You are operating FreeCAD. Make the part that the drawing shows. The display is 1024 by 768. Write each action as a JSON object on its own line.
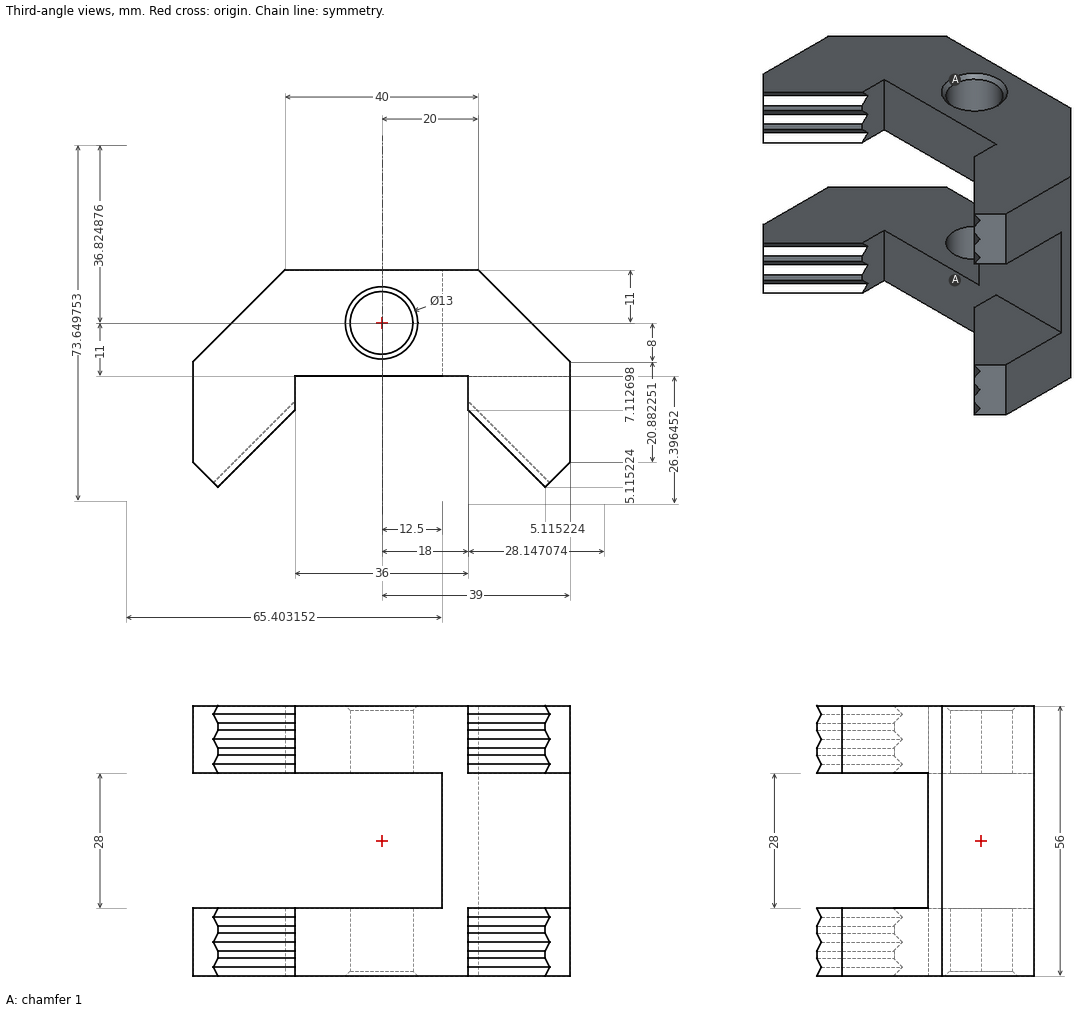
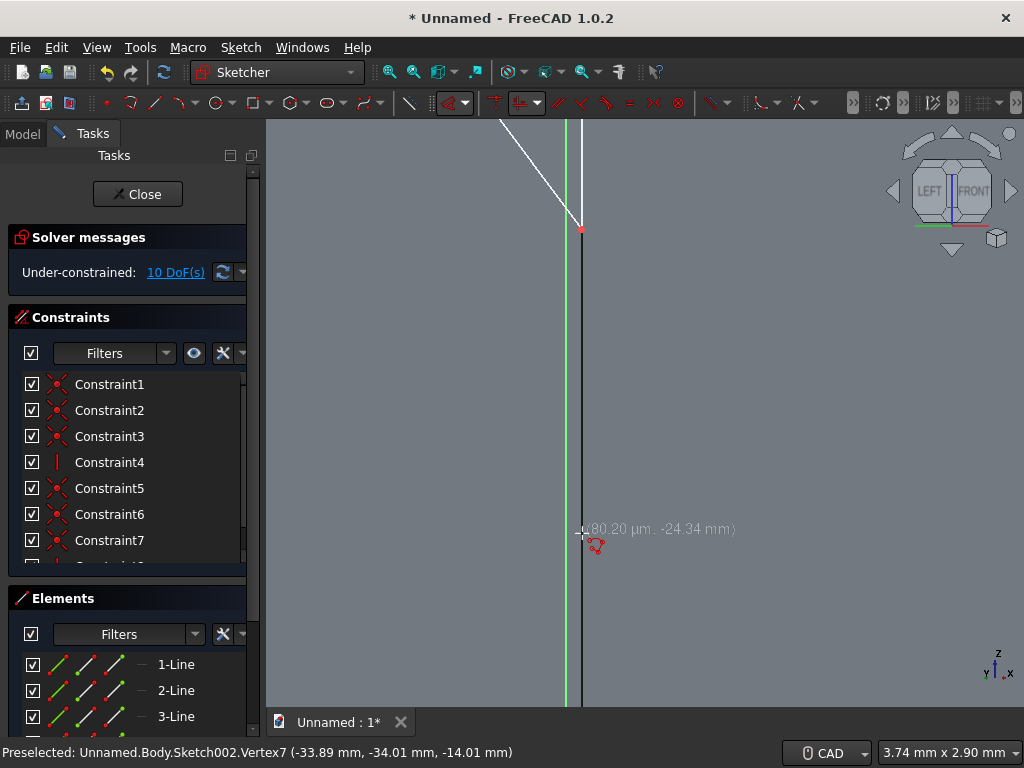
{"action": "scroll", "coordinate": [585, 541], "scroll_direction": "down", "scroll_amount": 14}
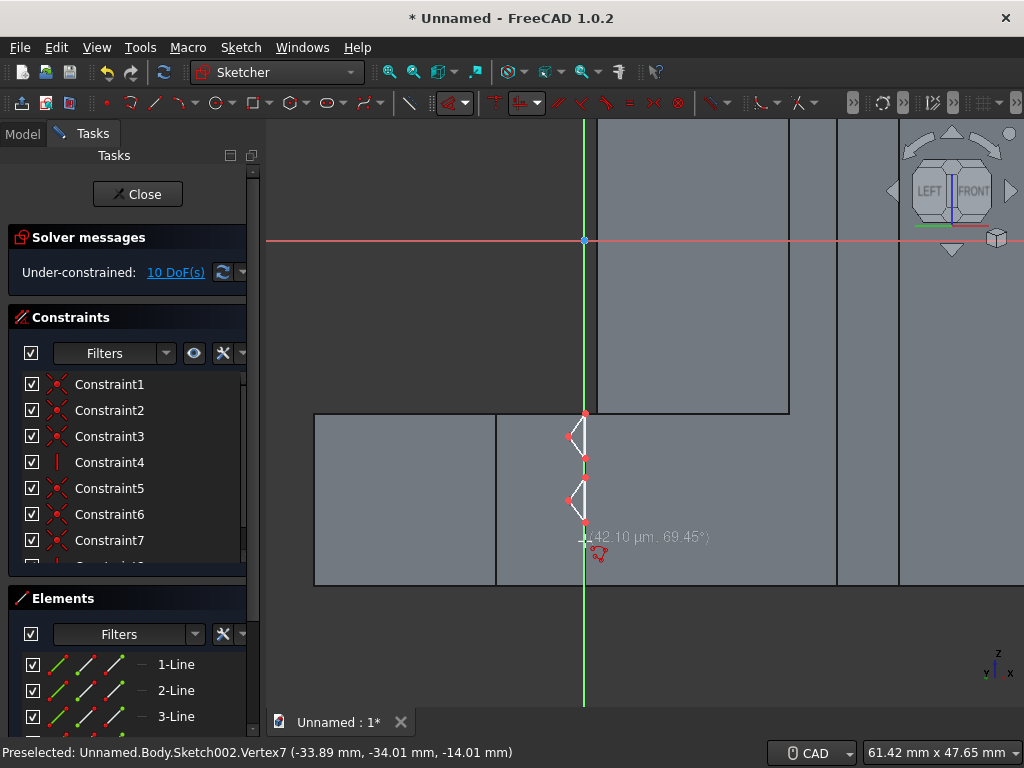
{"action": "left_click", "coordinate": [569, 564]}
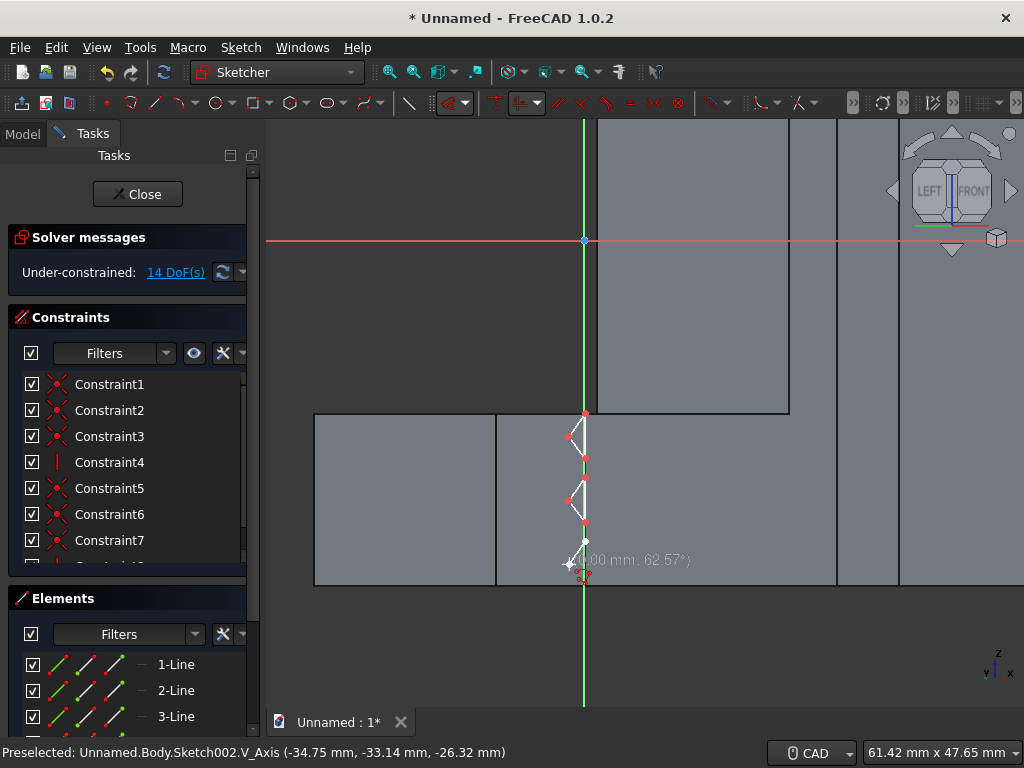
{"action": "scroll", "coordinate": [585, 586], "scroll_direction": "up", "scroll_amount": 14}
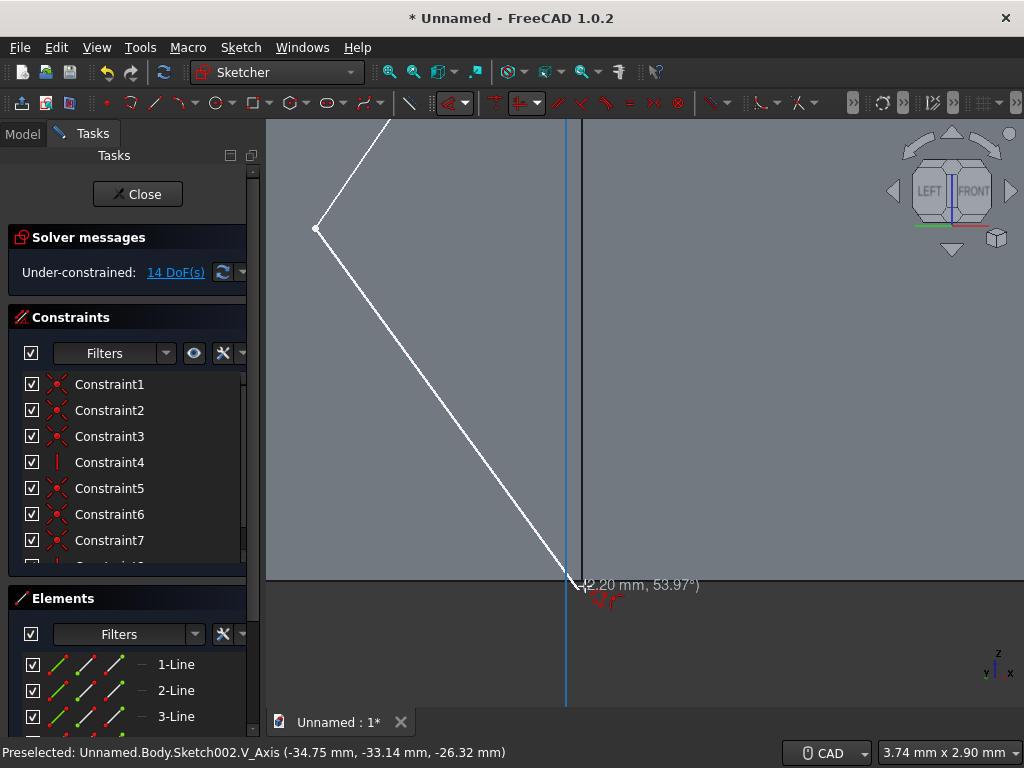
{"action": "left_click", "coordinate": [582, 581]}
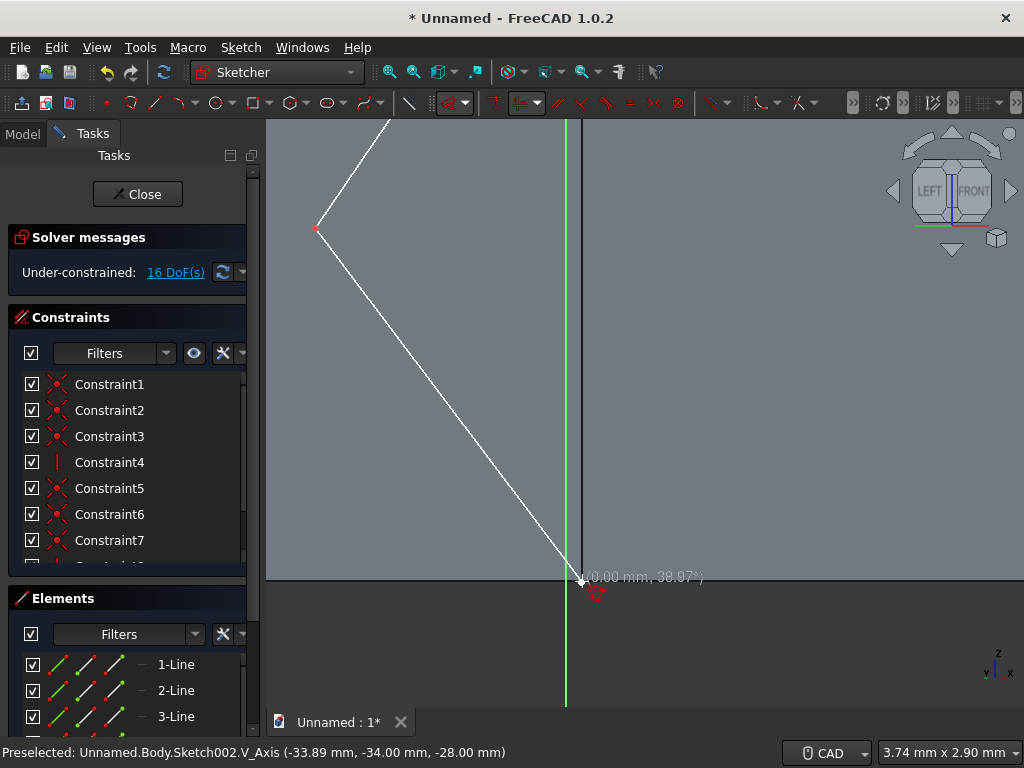
{"action": "scroll", "coordinate": [585, 586], "scroll_direction": "down", "scroll_amount": 14}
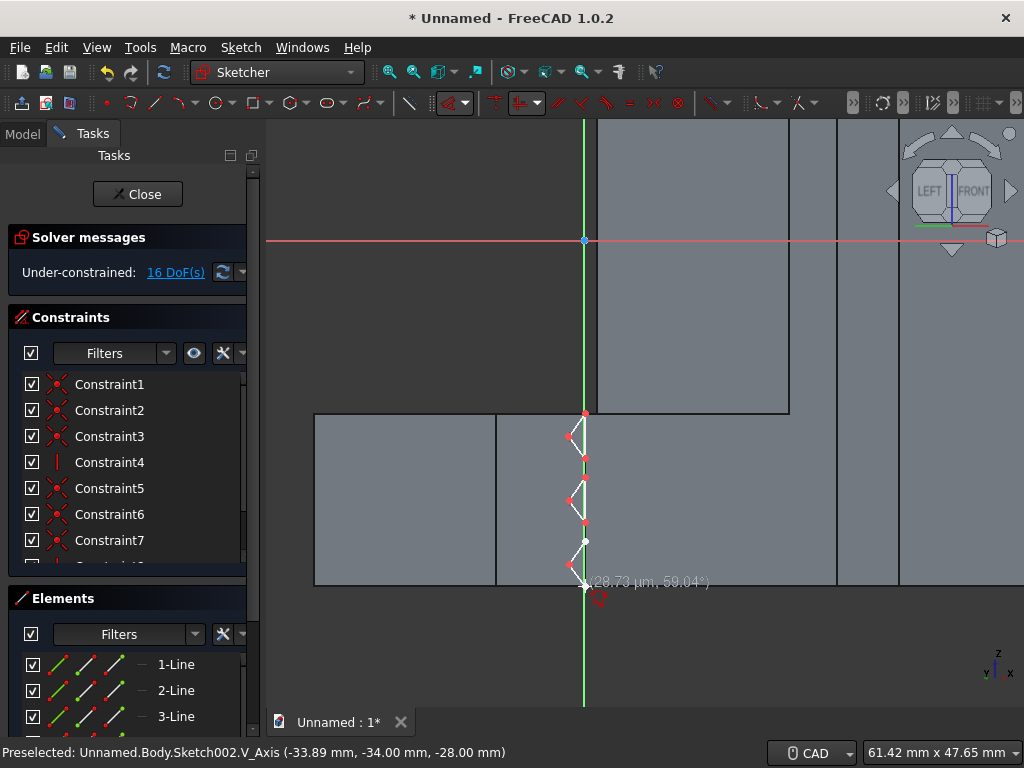
{"action": "scroll", "coordinate": [585, 541], "scroll_direction": "up", "scroll_amount": 14}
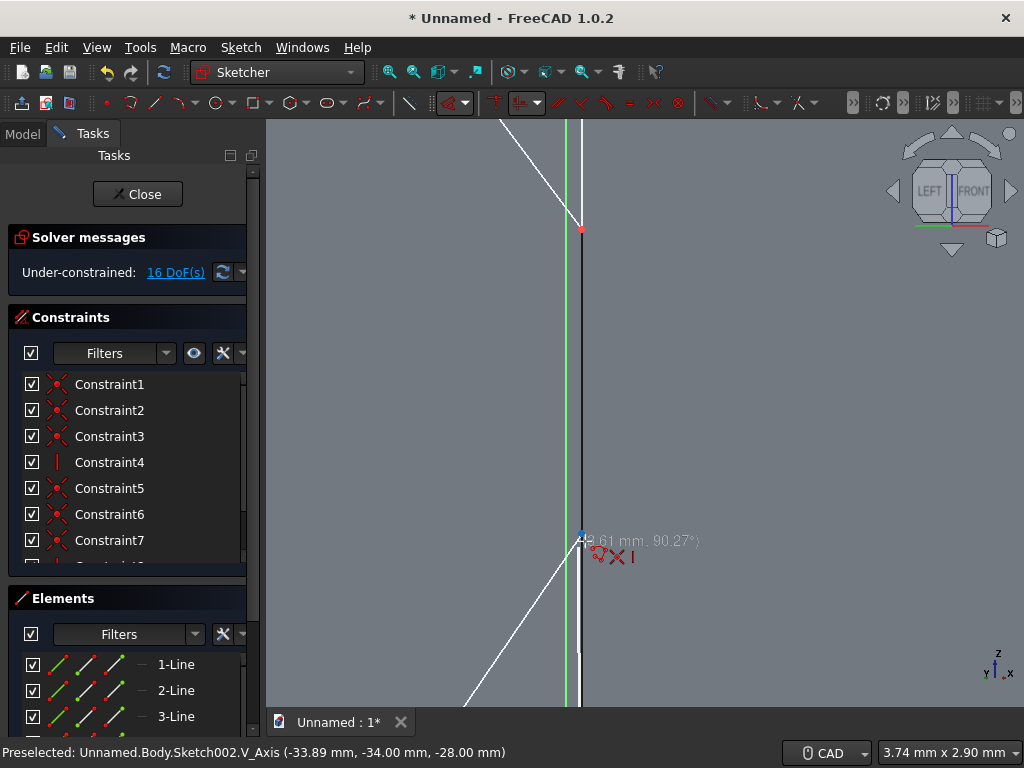
{"action": "left_click", "coordinate": [582, 534]}
{"action": "key", "text": "Escape"}
{"action": "key", "text": "Escape"}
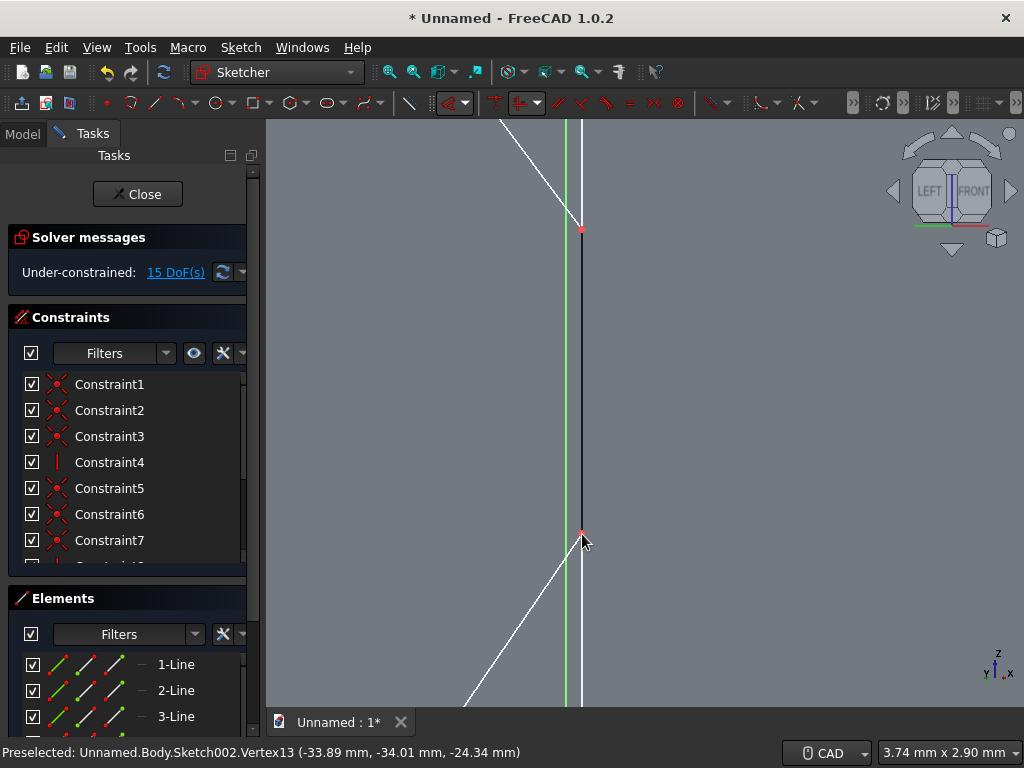
{"action": "scroll", "coordinate": [585, 541], "scroll_direction": "down", "scroll_amount": 14}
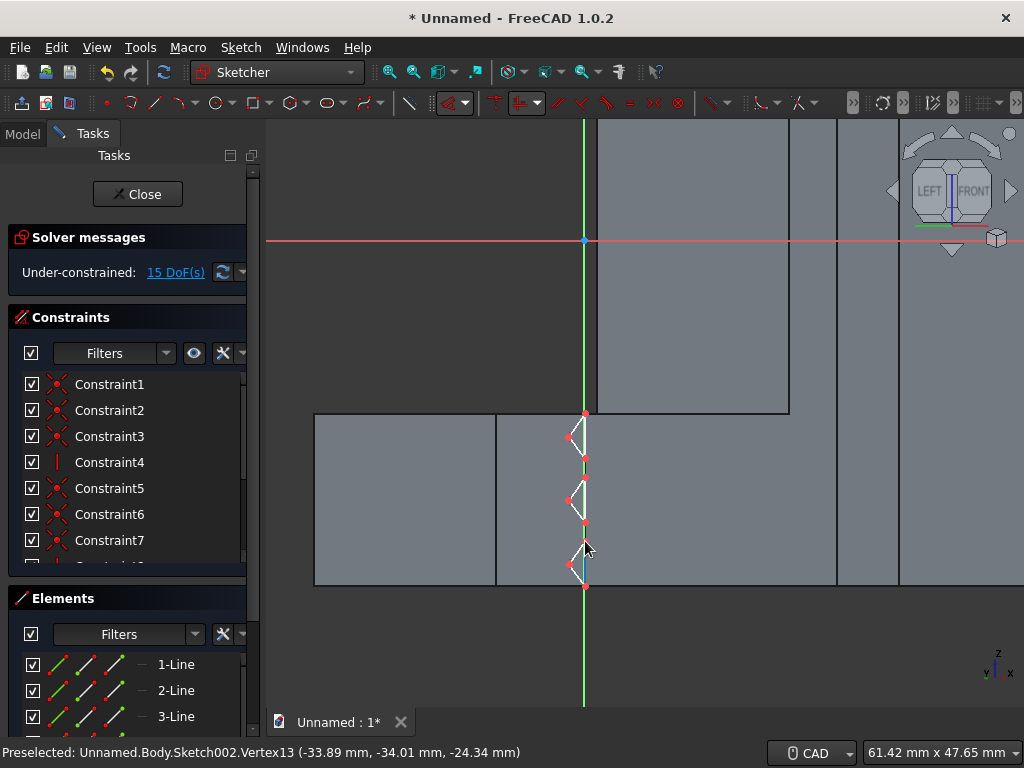
{"action": "left_click", "coordinate": [569, 501]}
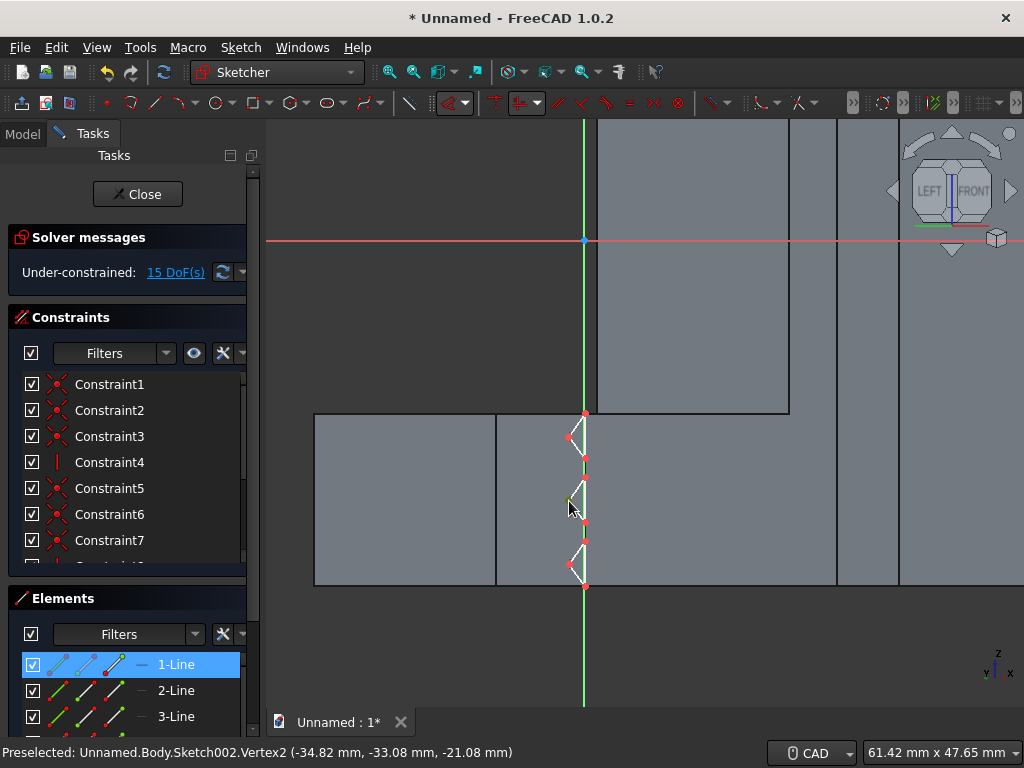
{"action": "left_click", "coordinate": [468, 104]}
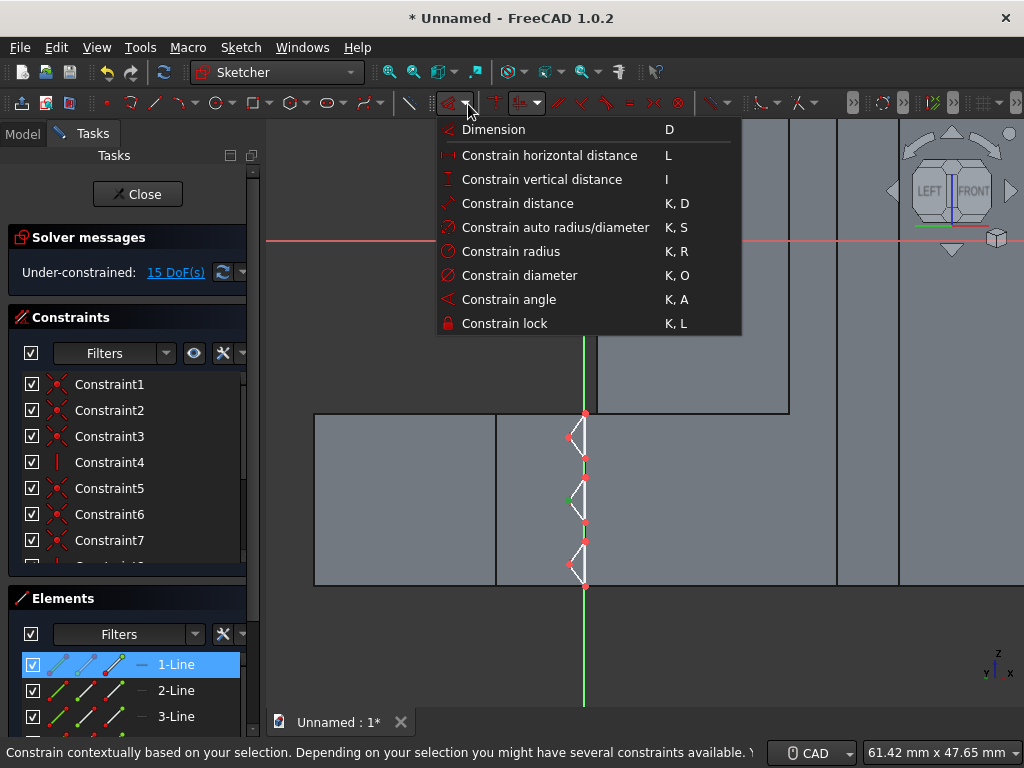
{"action": "left_click", "coordinate": [589, 179]}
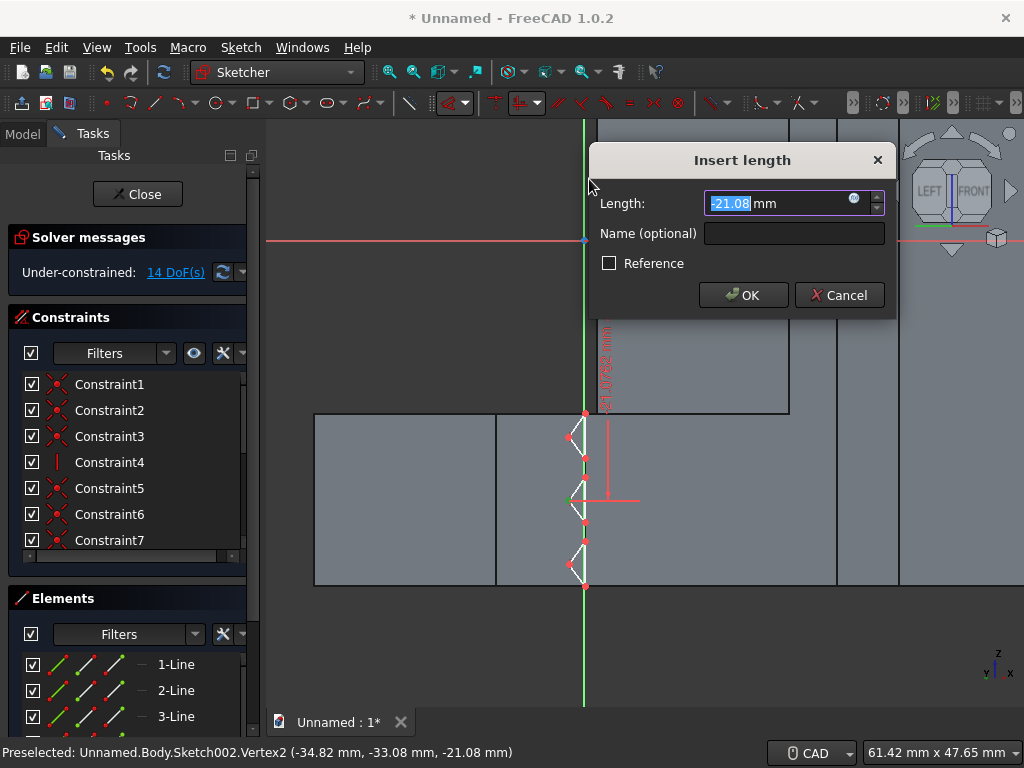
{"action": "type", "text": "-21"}
{"action": "key", "text": "Return"}